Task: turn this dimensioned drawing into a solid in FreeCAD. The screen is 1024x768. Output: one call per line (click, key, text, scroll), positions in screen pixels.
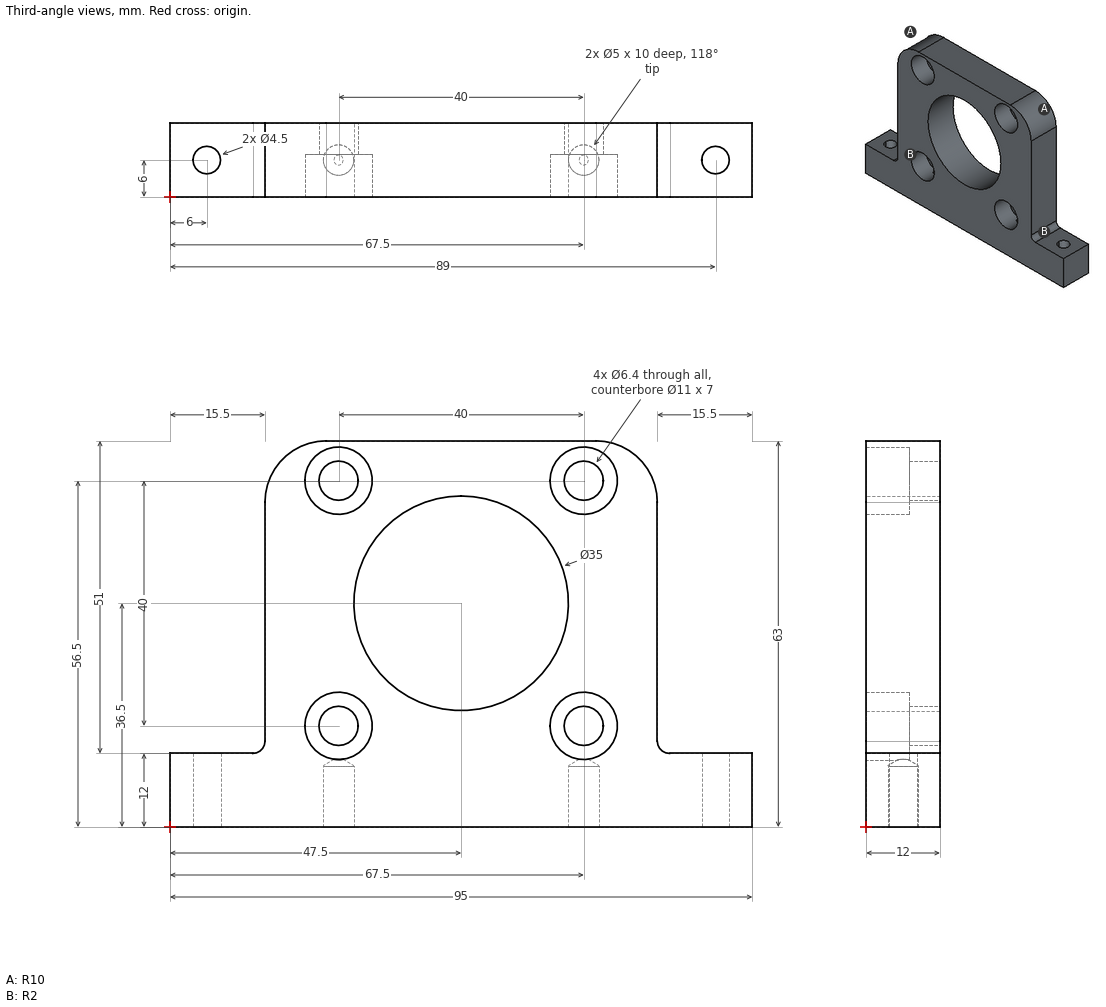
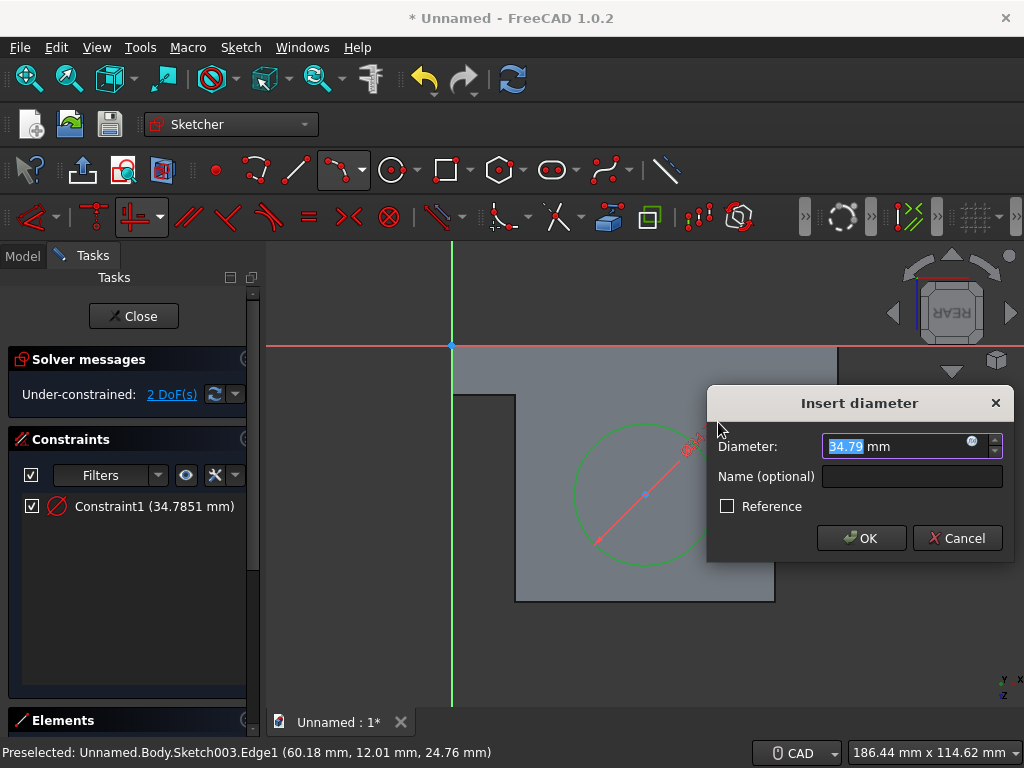
text(35)
key(Return)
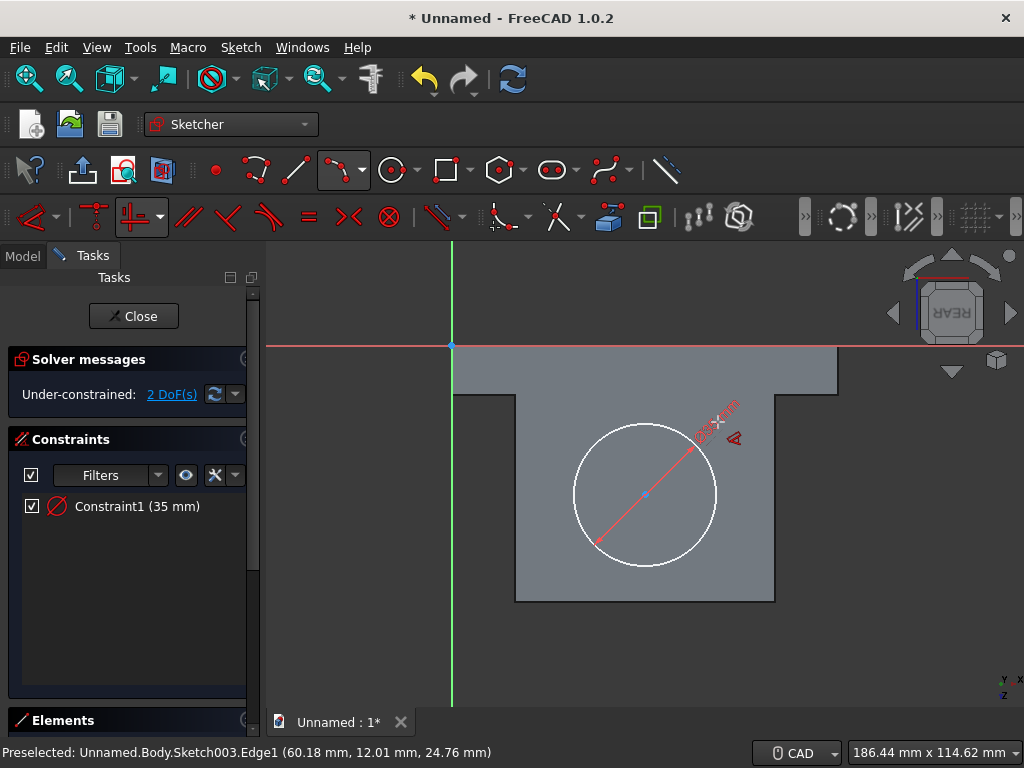
click(645, 495)
click(548, 312)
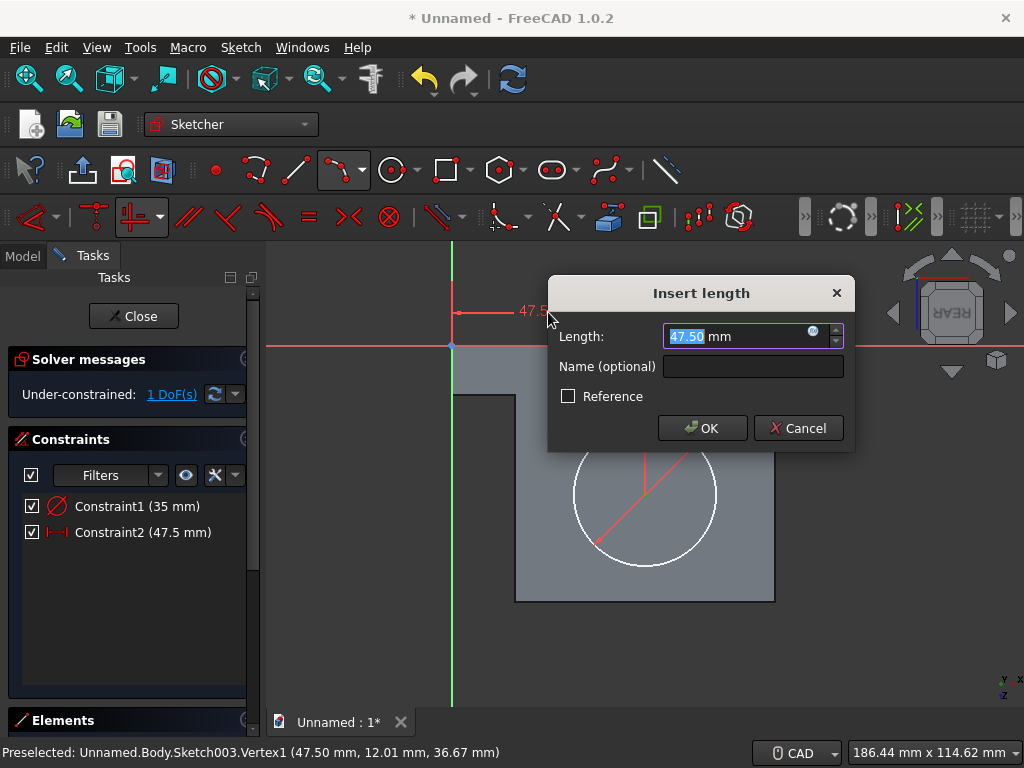
text(47.5)
key(Return)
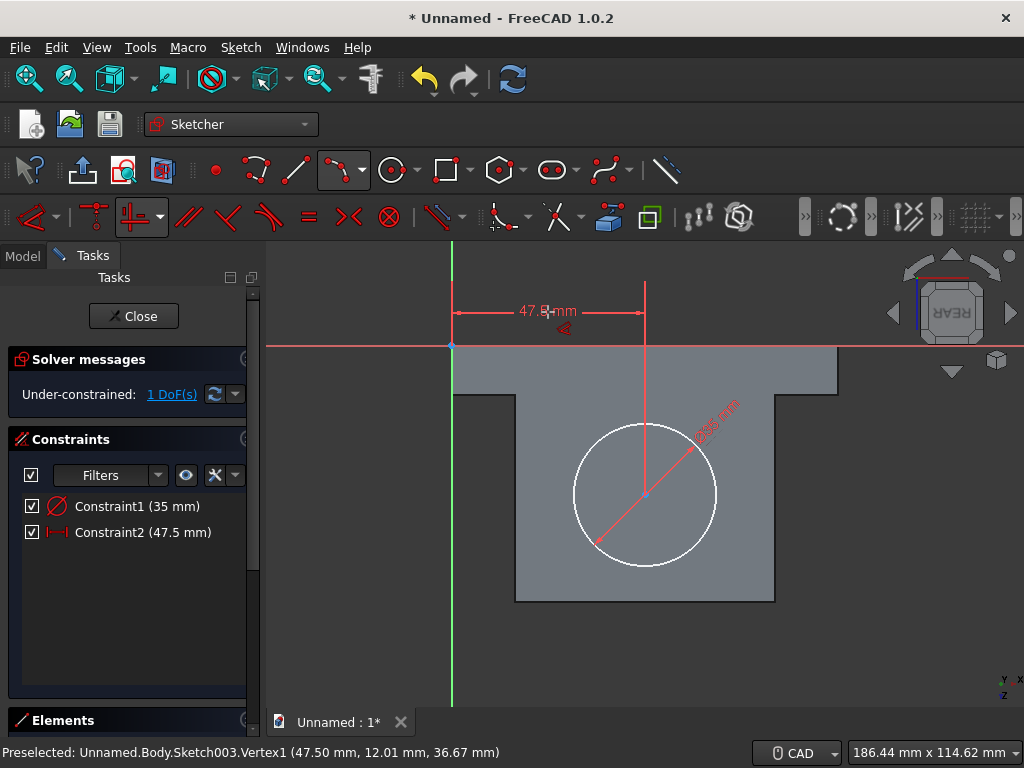
click(645, 495)
click(418, 420)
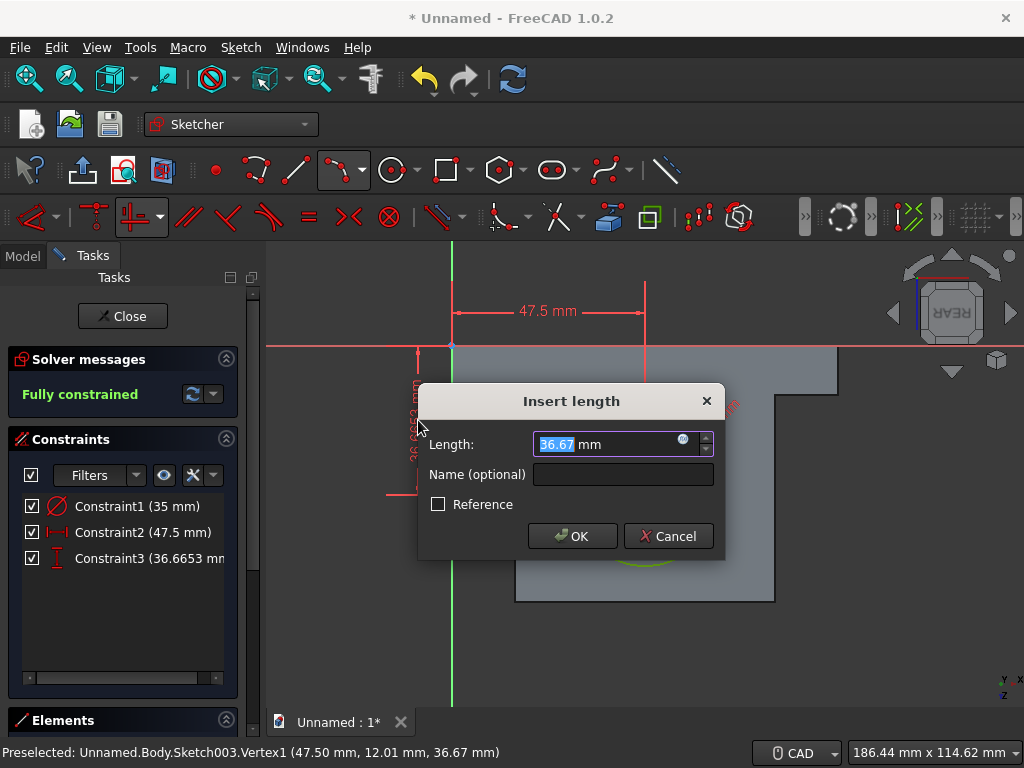
text(36.5)
key(Return)
key(Escape)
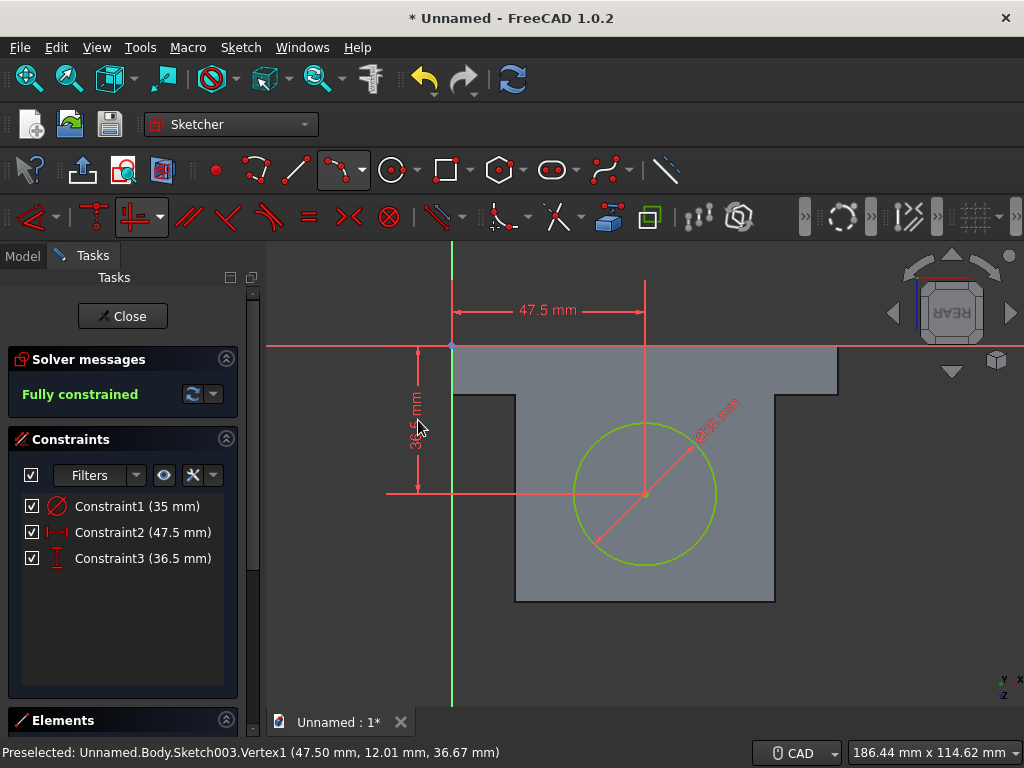
click(123, 316)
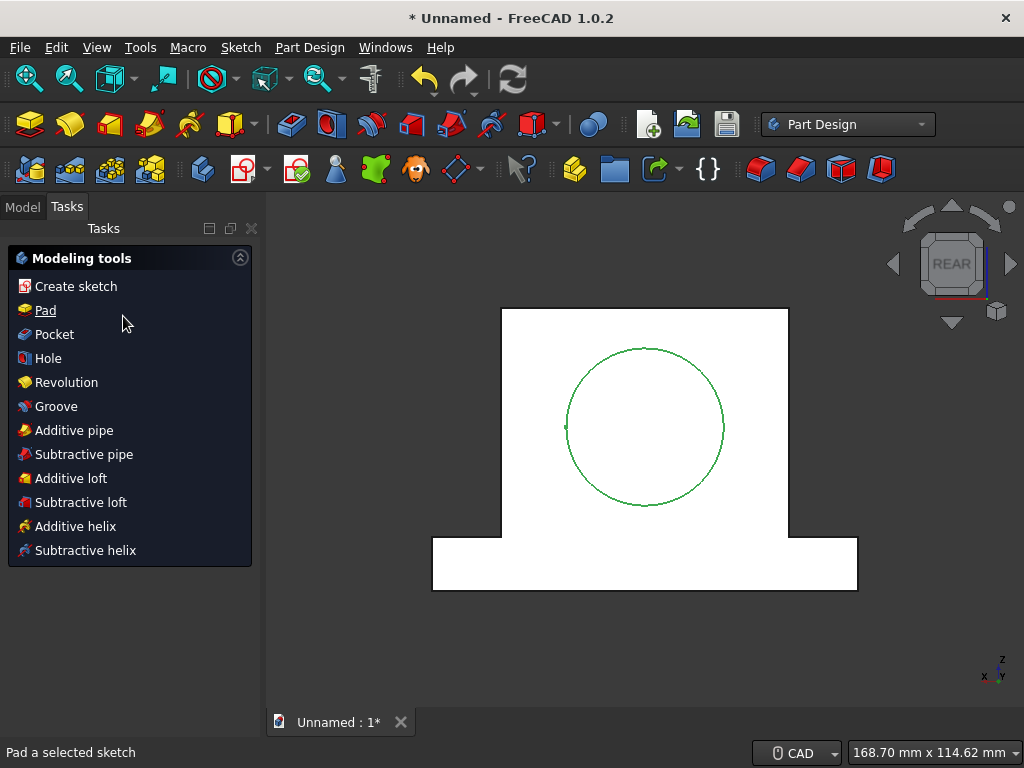
click(292, 124)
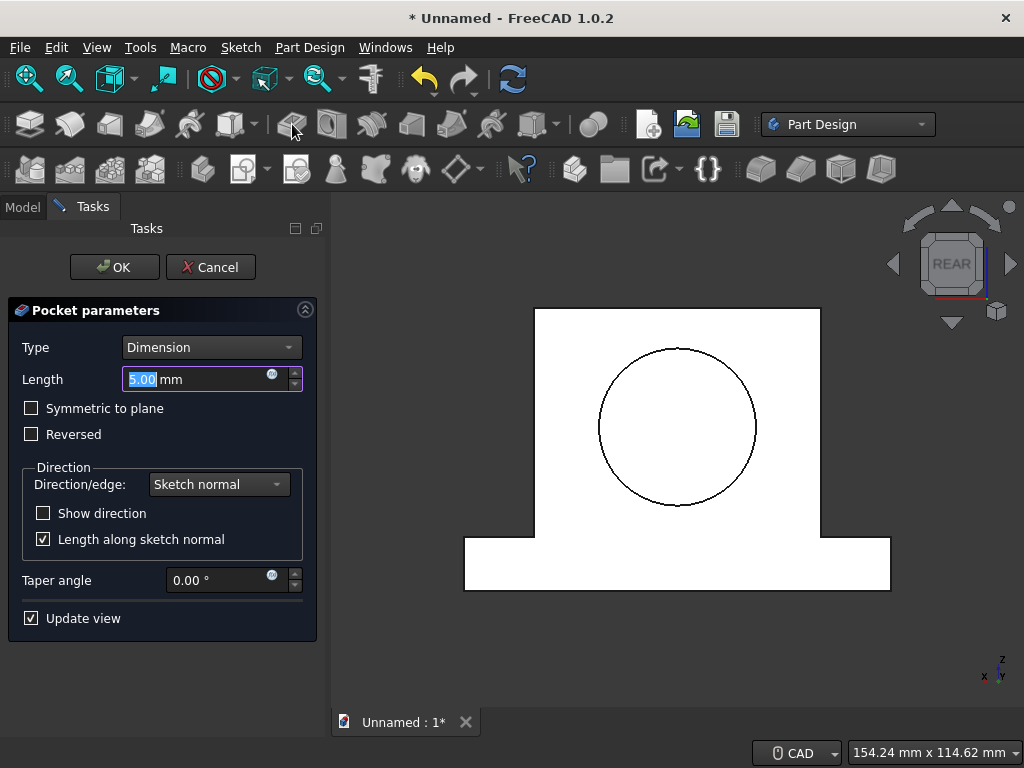
click(212, 348)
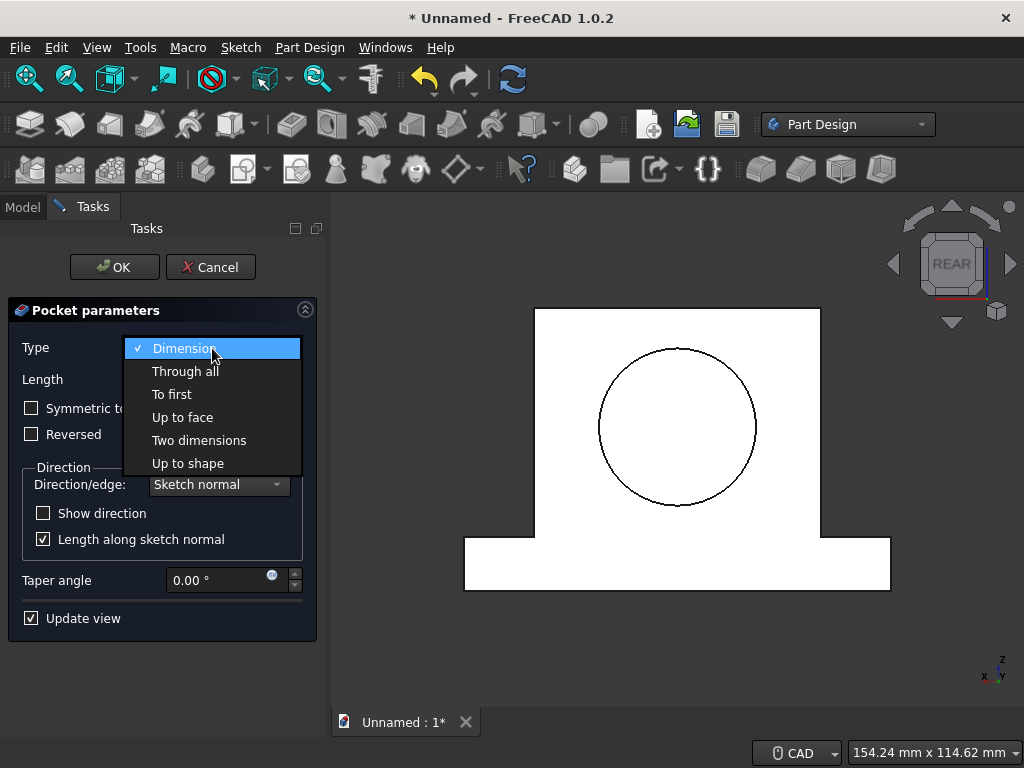
click(212, 372)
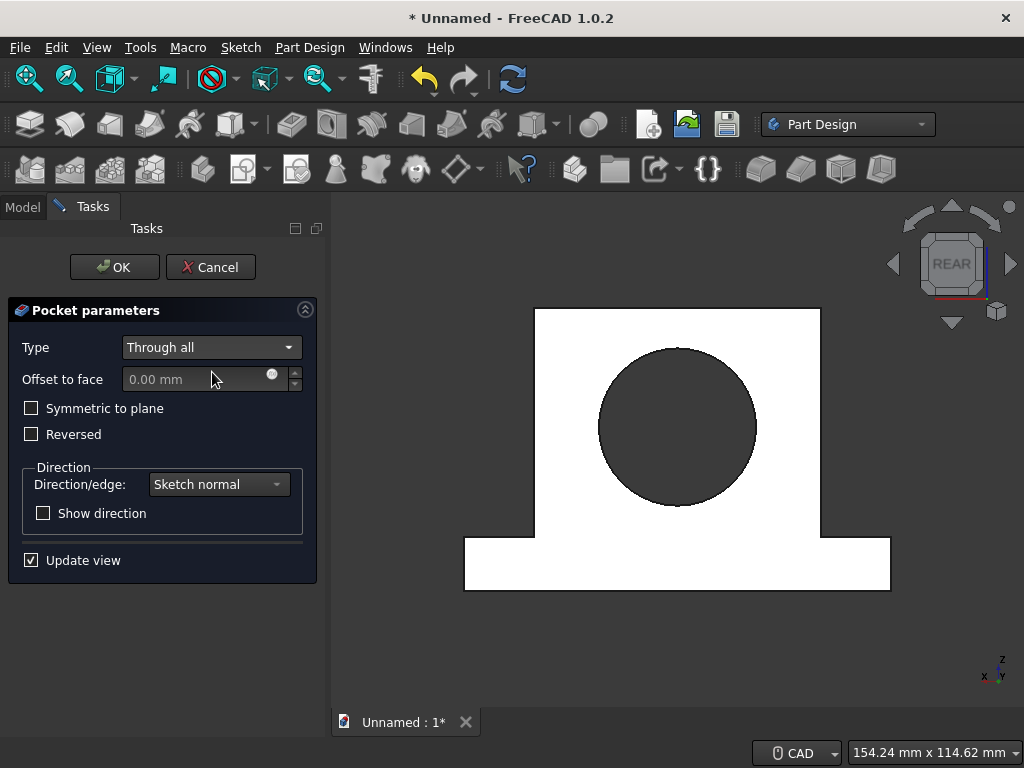
click(115, 267)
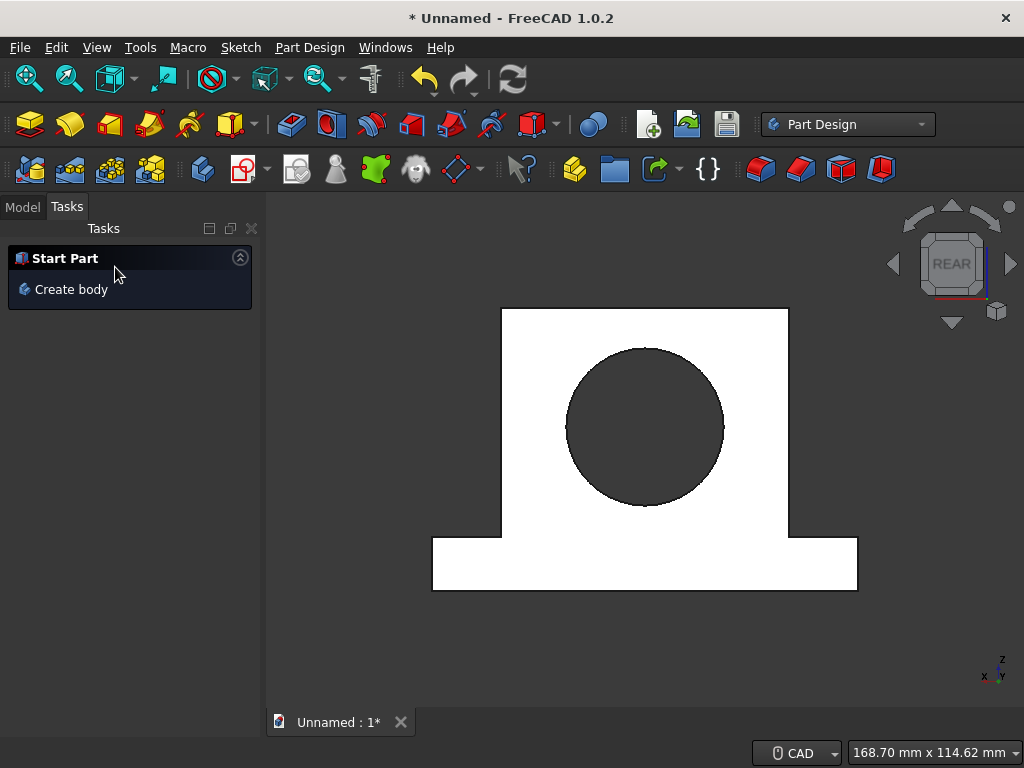
key(0)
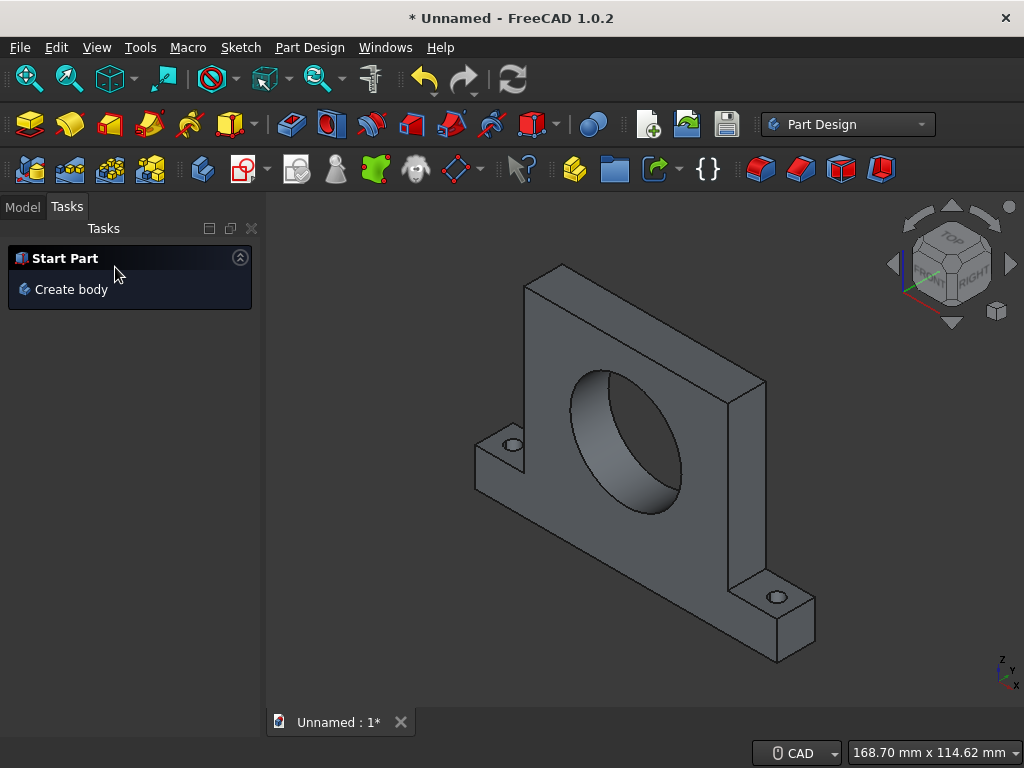
click(747, 392)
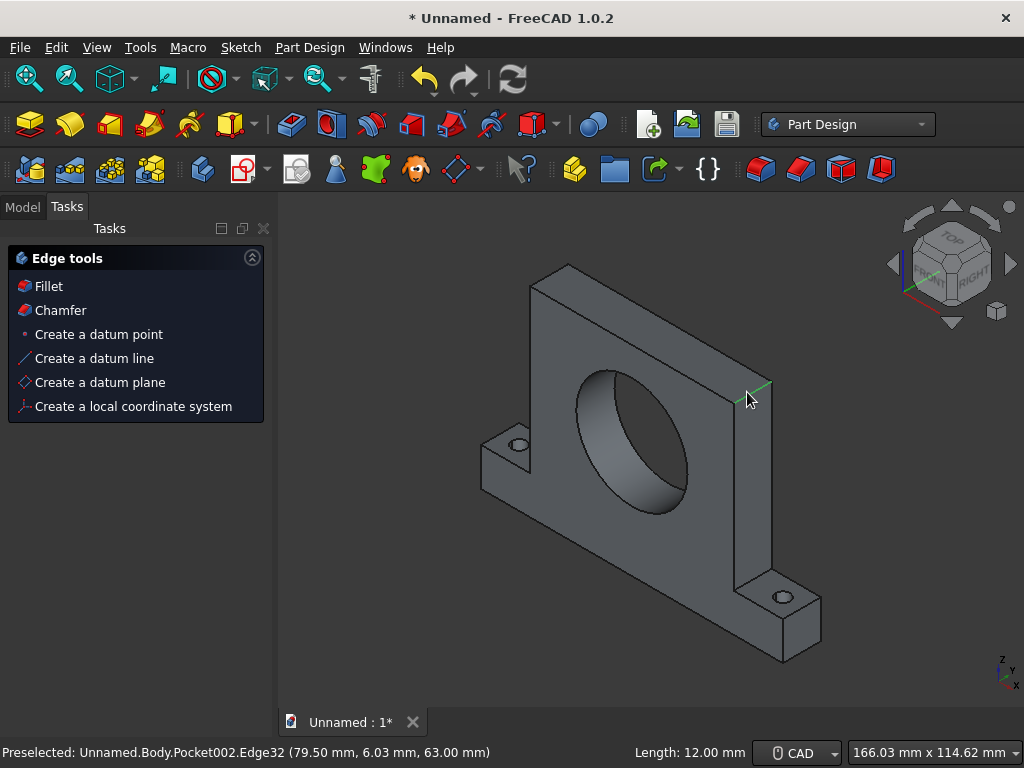
key(2)